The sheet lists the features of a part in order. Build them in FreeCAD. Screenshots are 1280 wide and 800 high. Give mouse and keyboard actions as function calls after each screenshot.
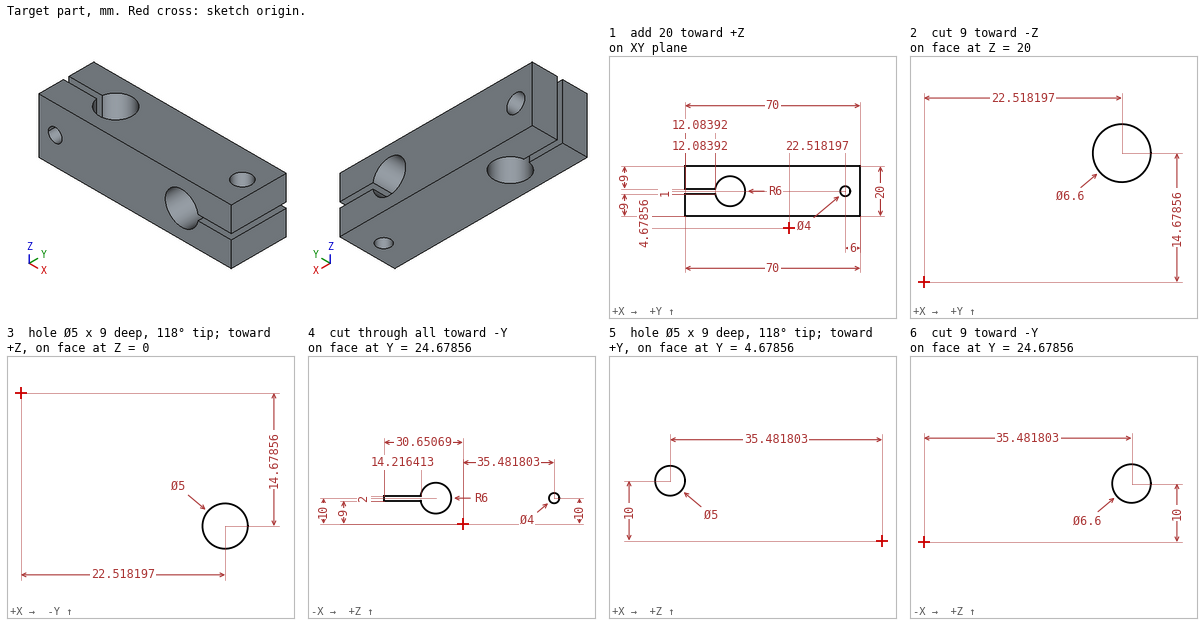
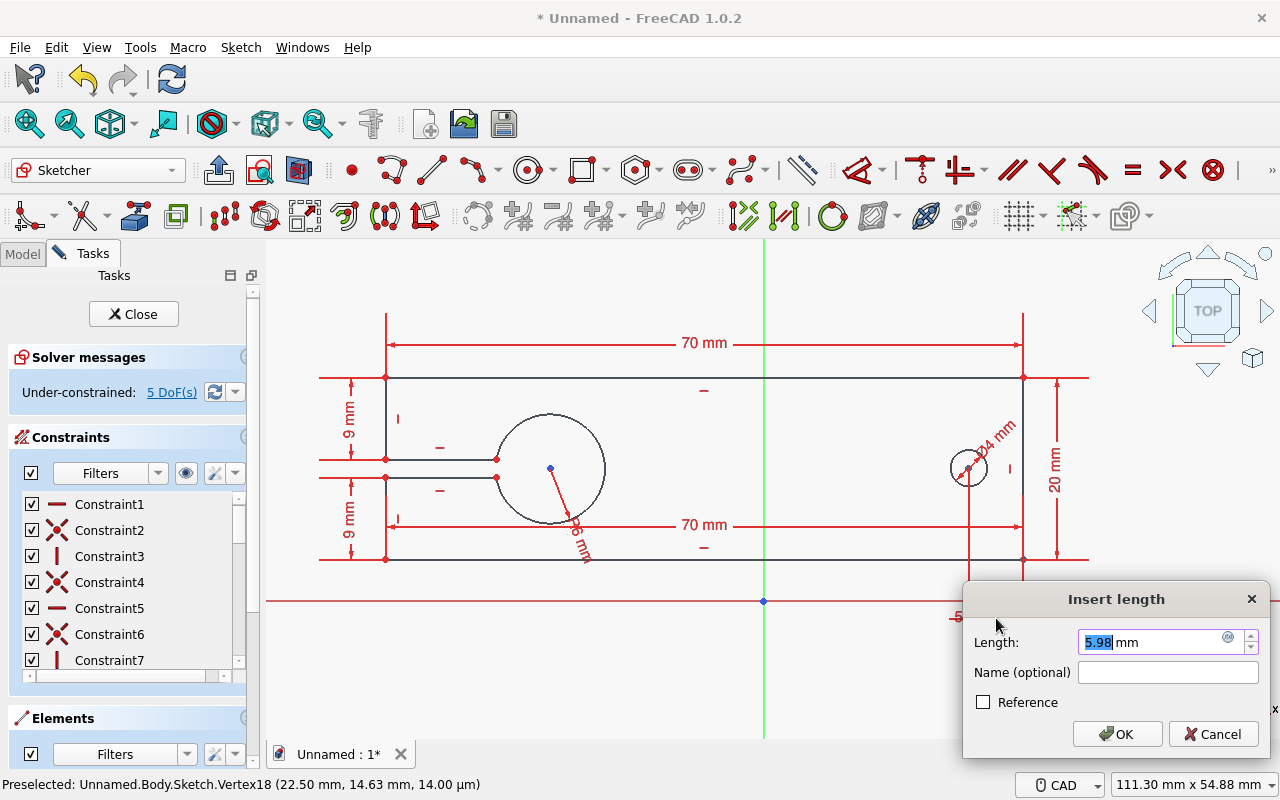
text(6)
key(Return)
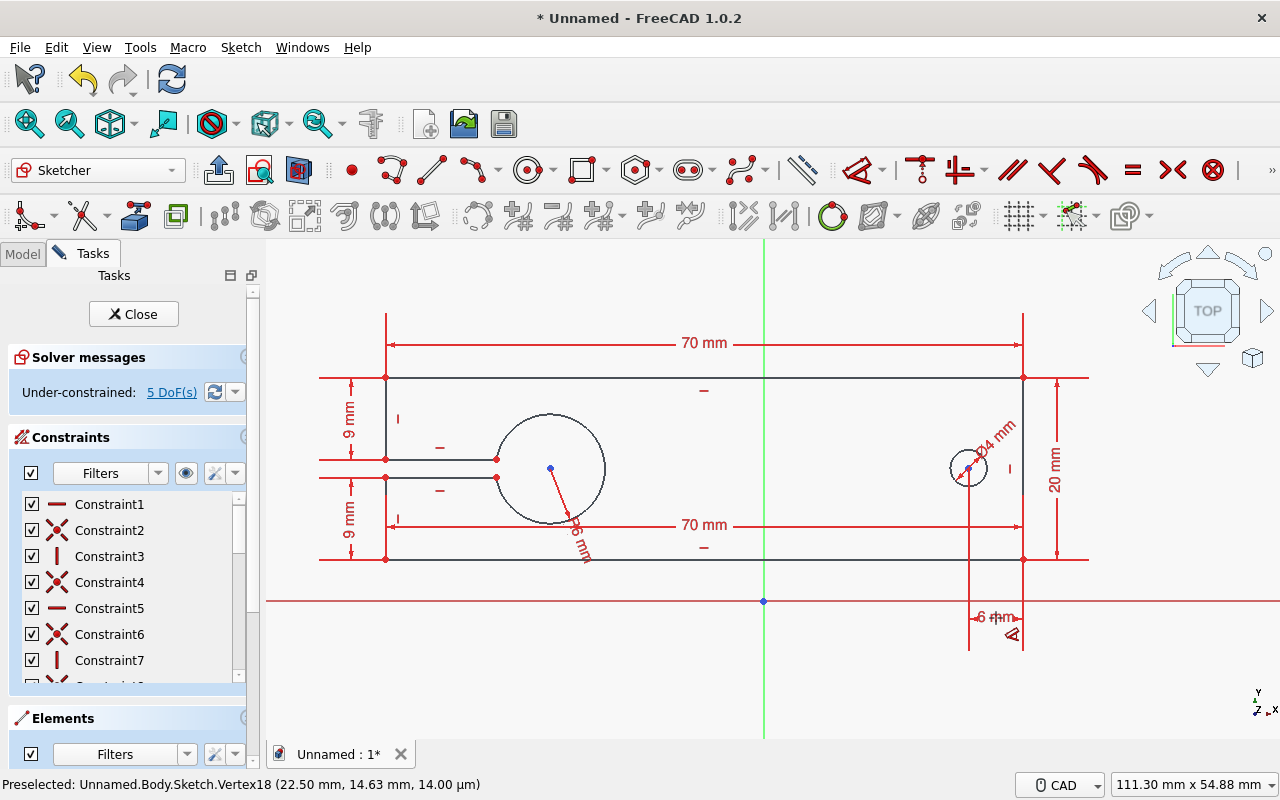
scroll(496, 478, up, 8)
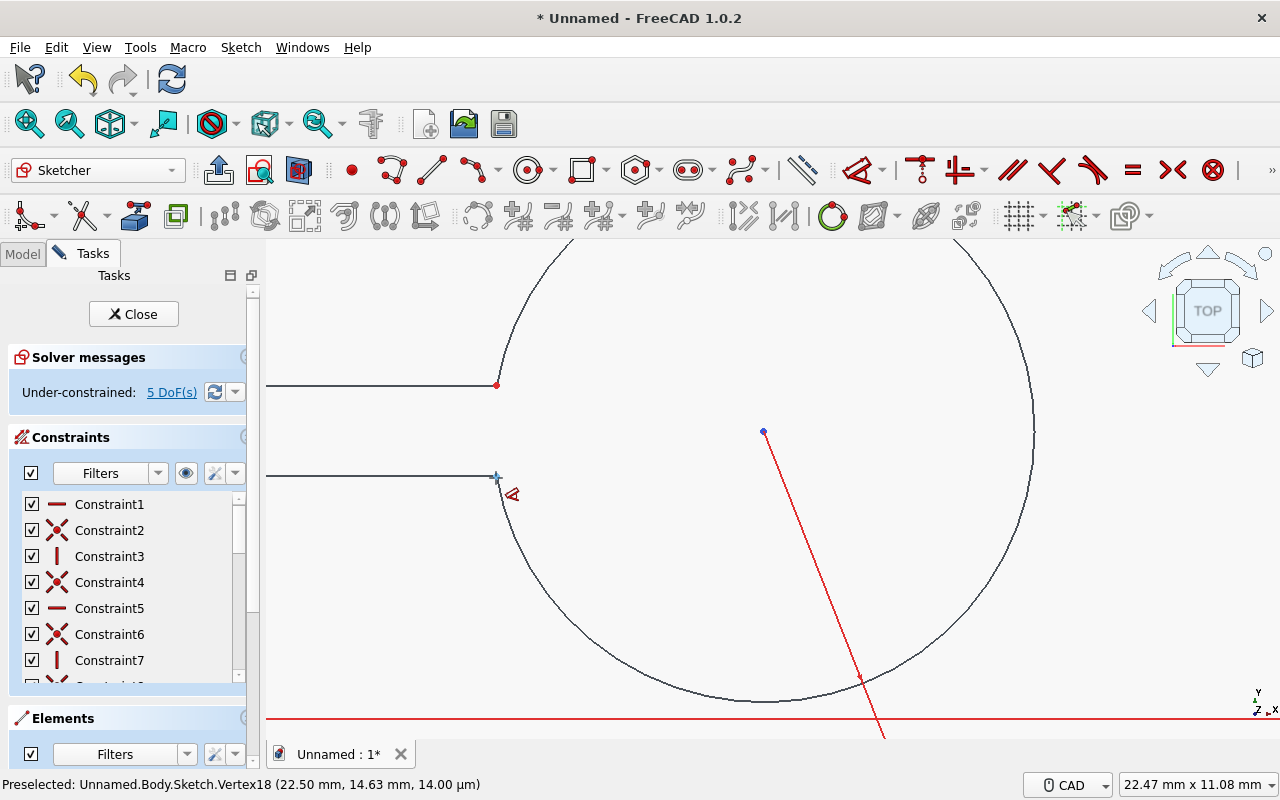
click(497, 476)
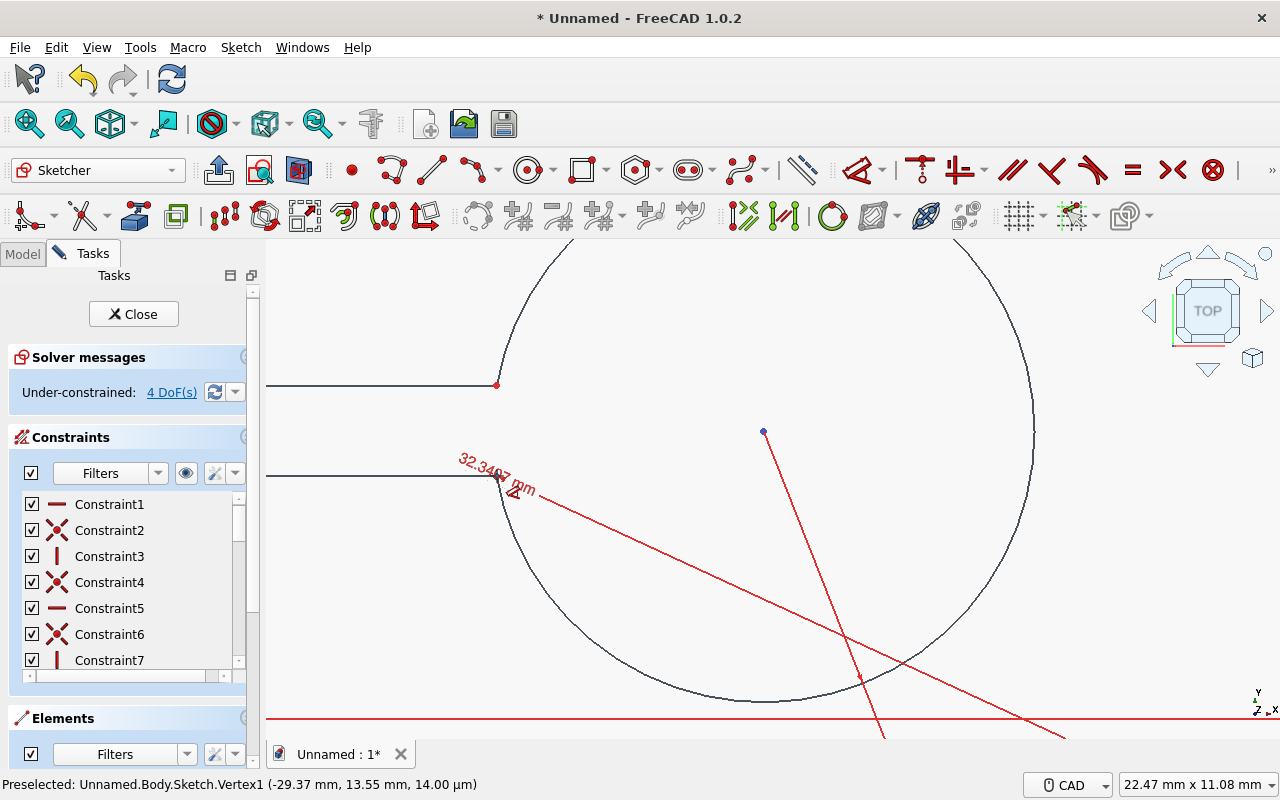
scroll(496, 478, down, 8)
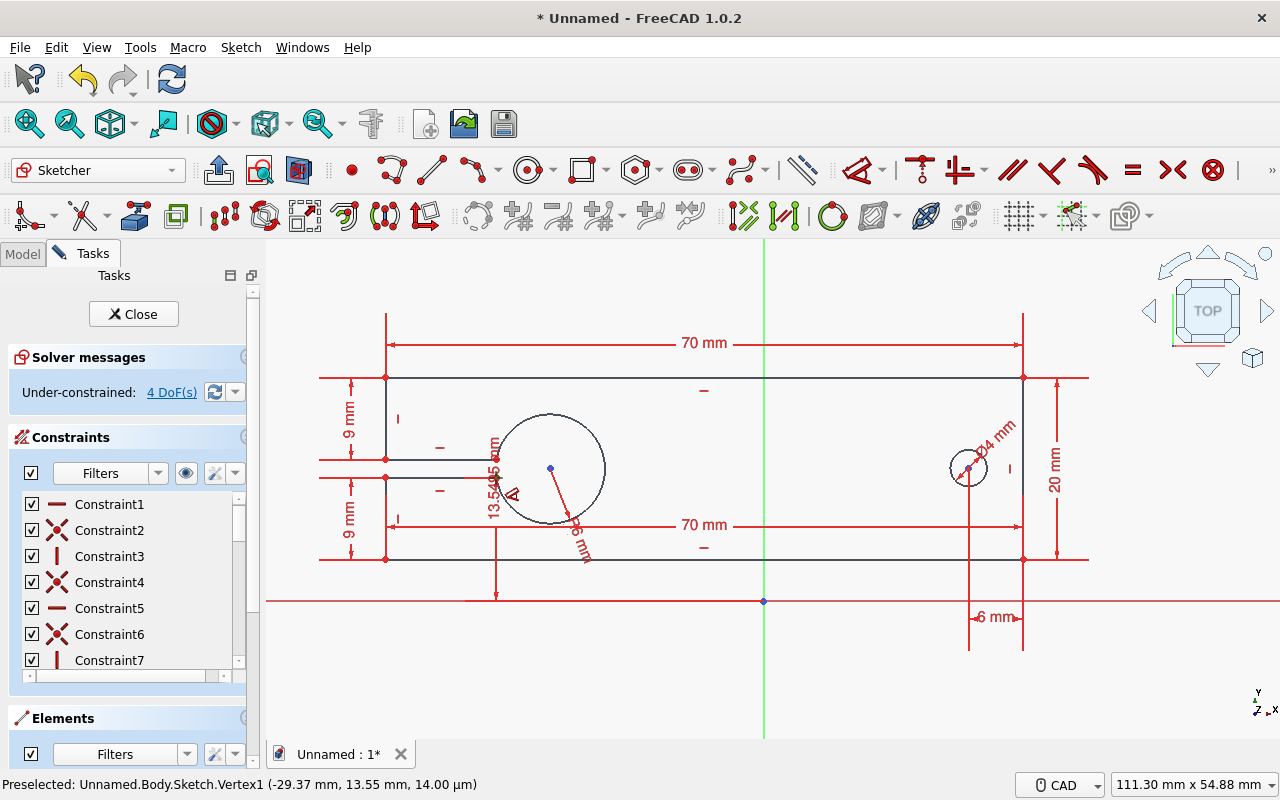
scroll(969, 468, up, 8)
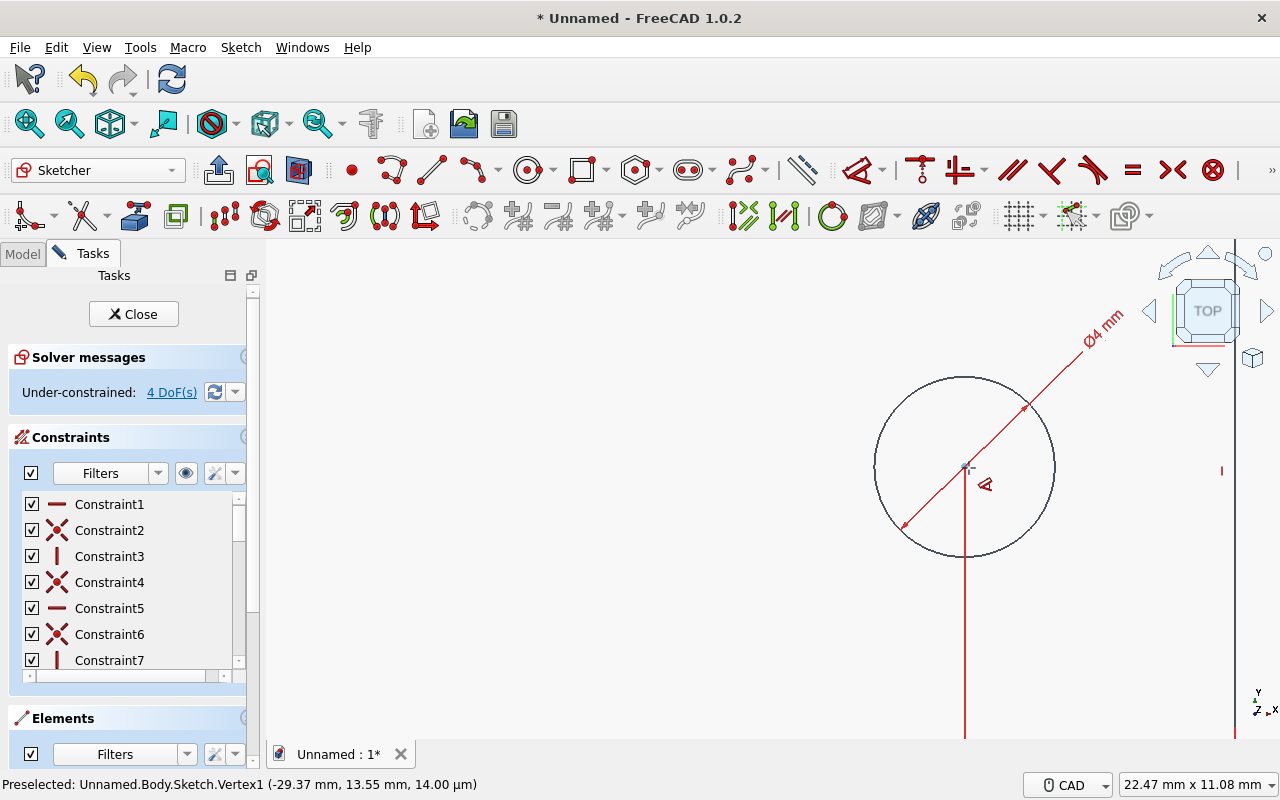
click(965, 467)
click(999, 491)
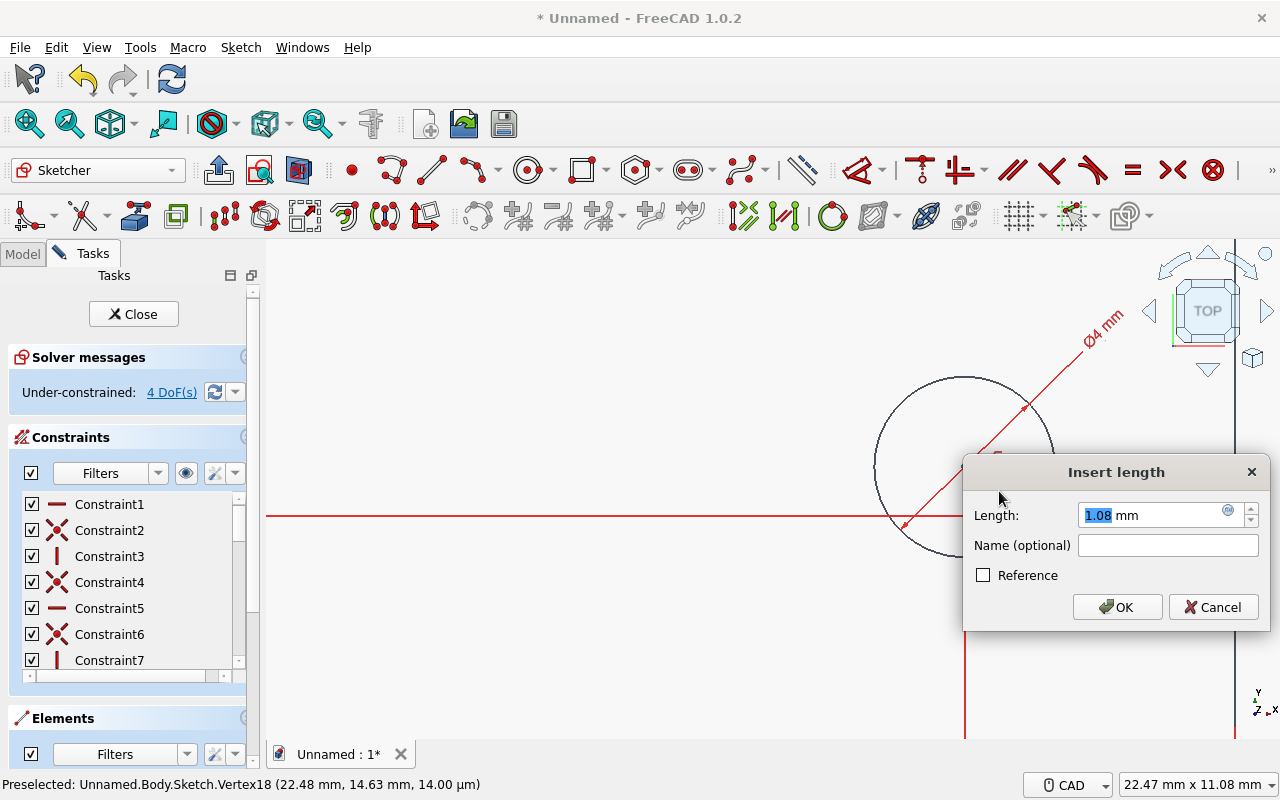
text(1)
key(Return)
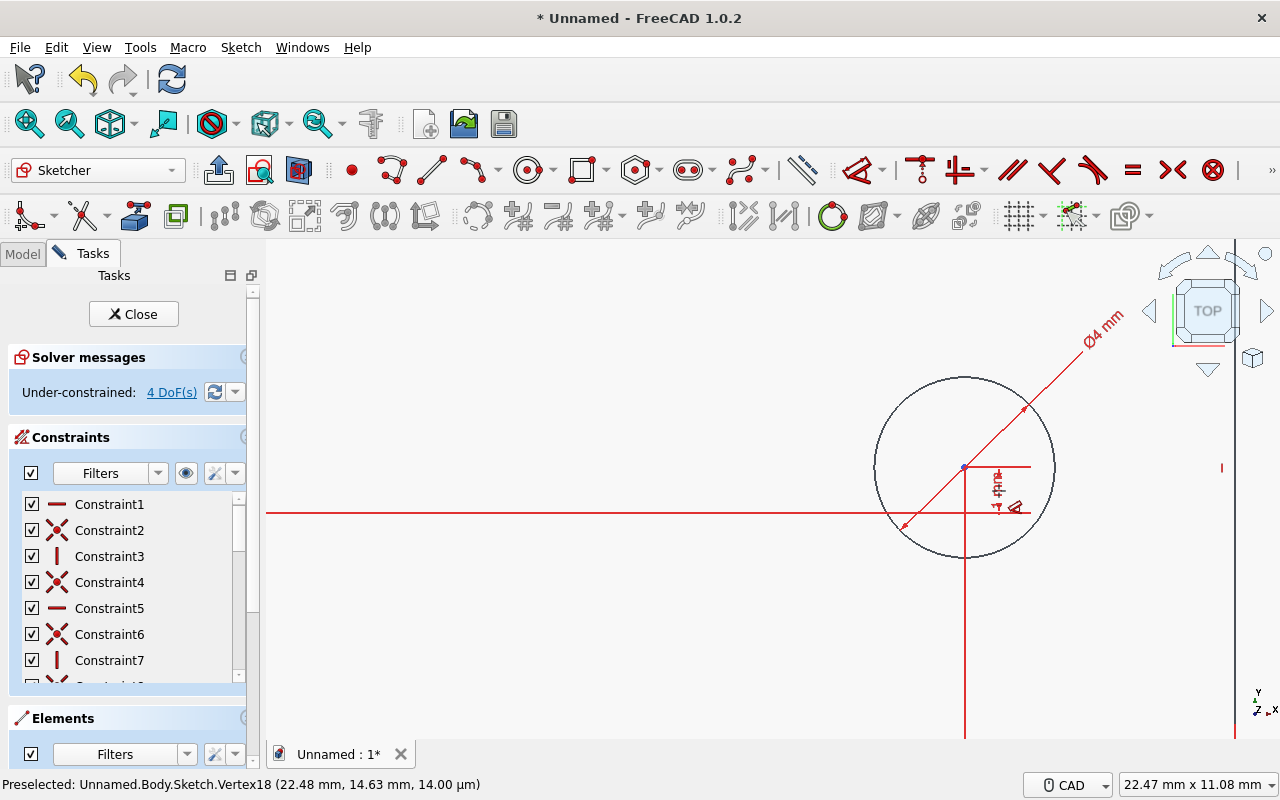
scroll(969, 468, down, 8)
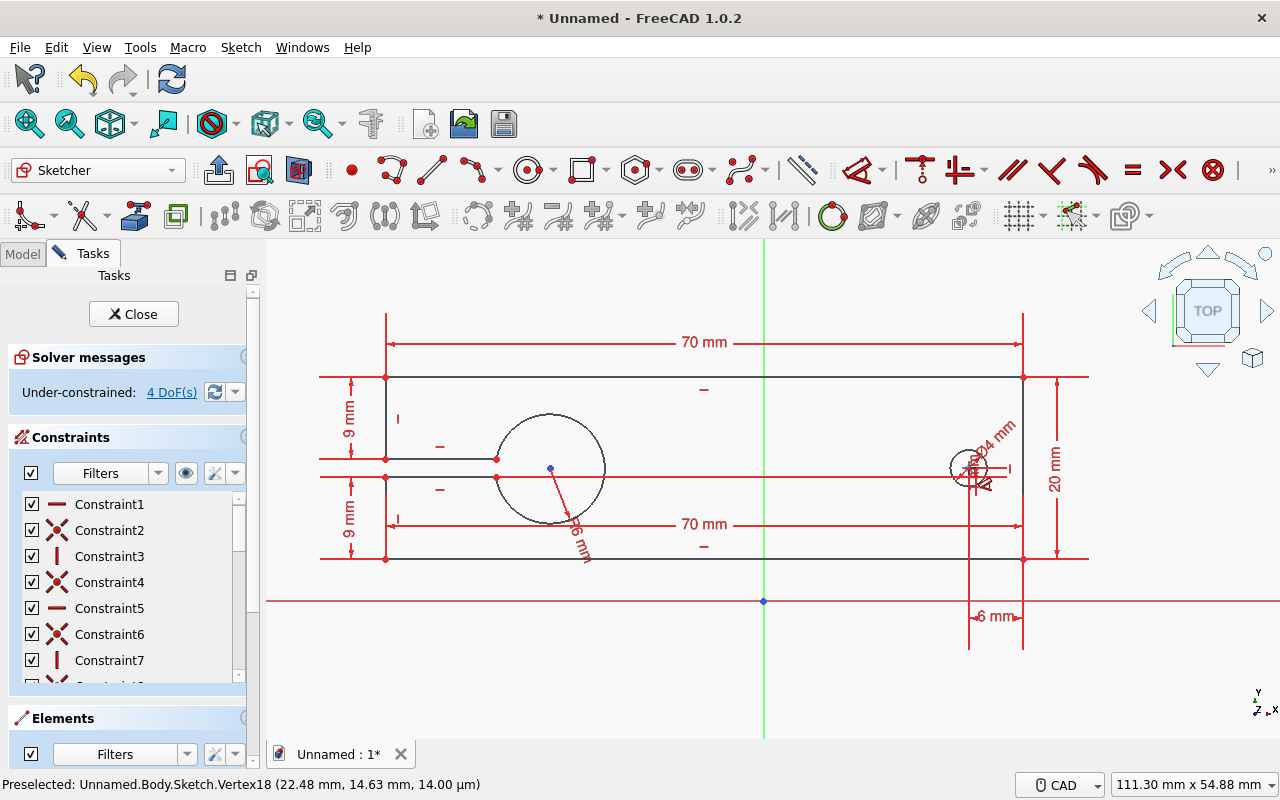
click(463, 477)
click(441, 443)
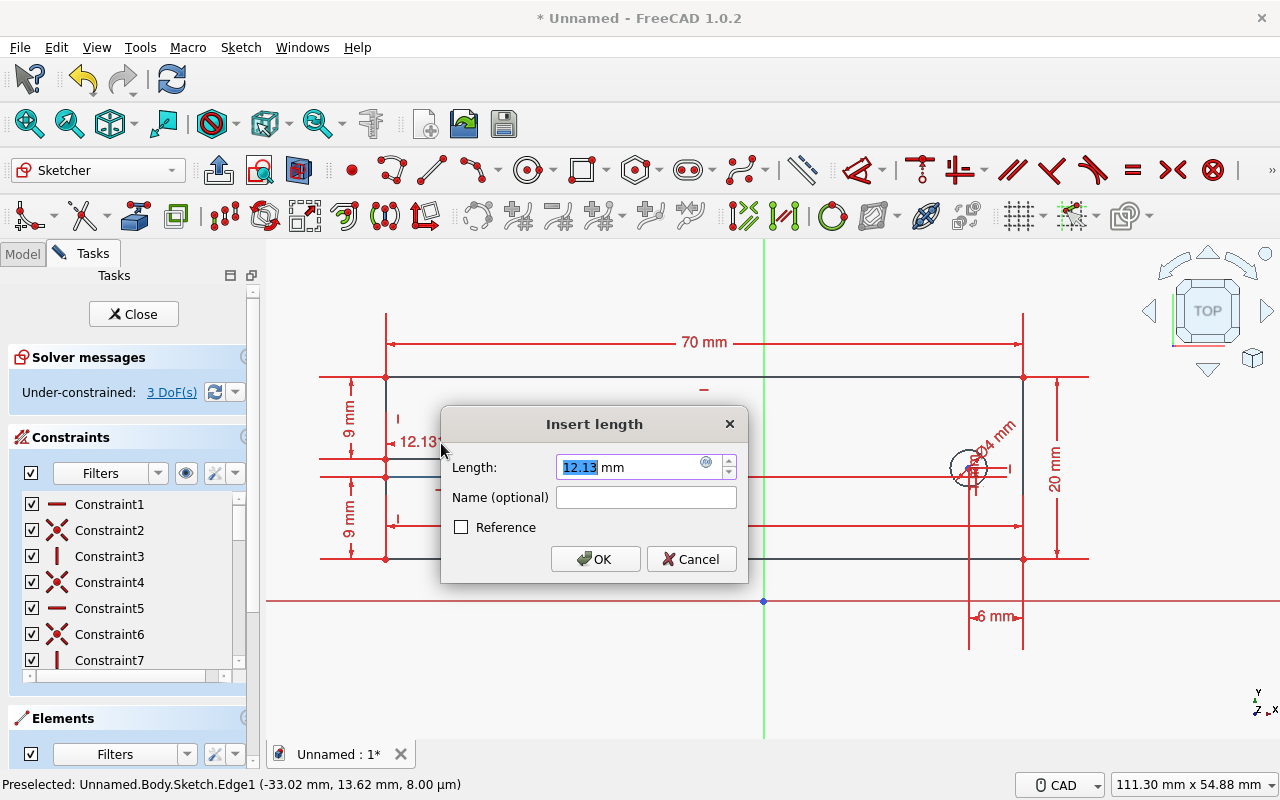
text(12.08392)
key(Return)